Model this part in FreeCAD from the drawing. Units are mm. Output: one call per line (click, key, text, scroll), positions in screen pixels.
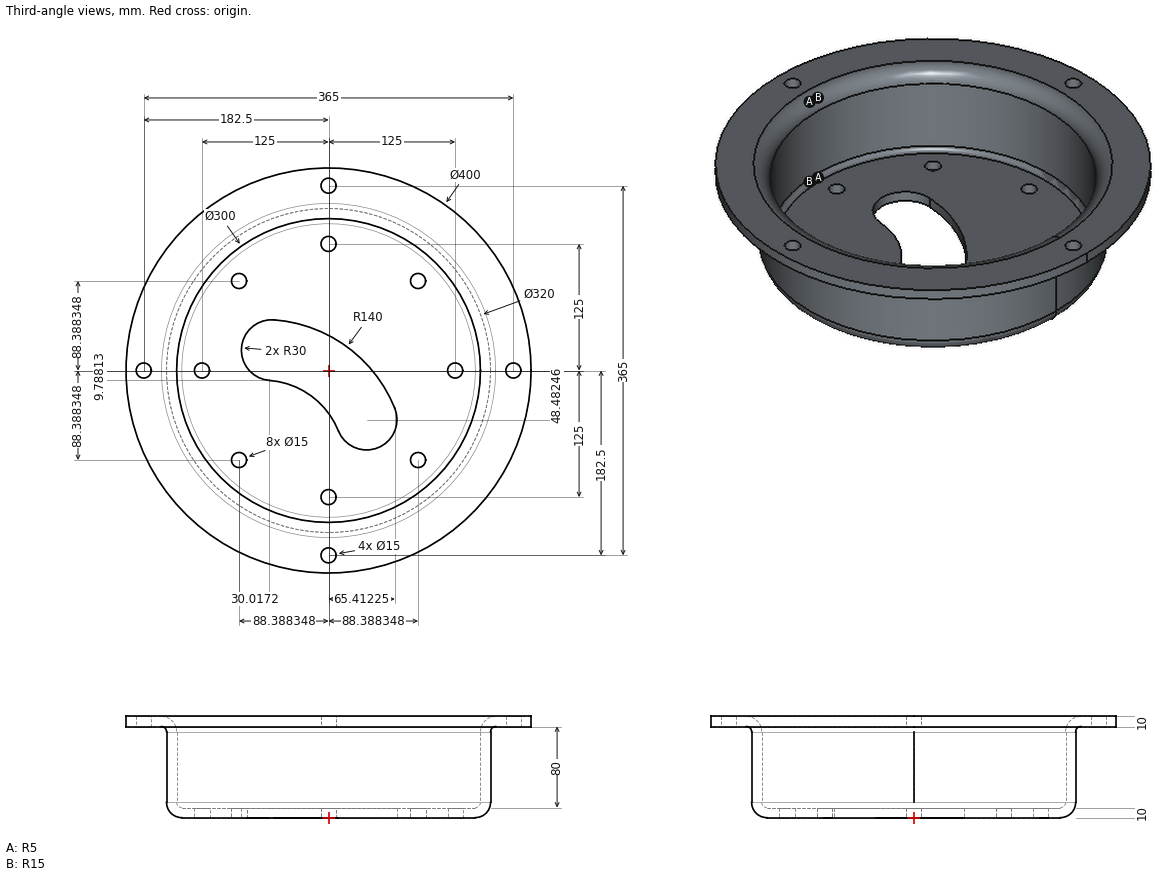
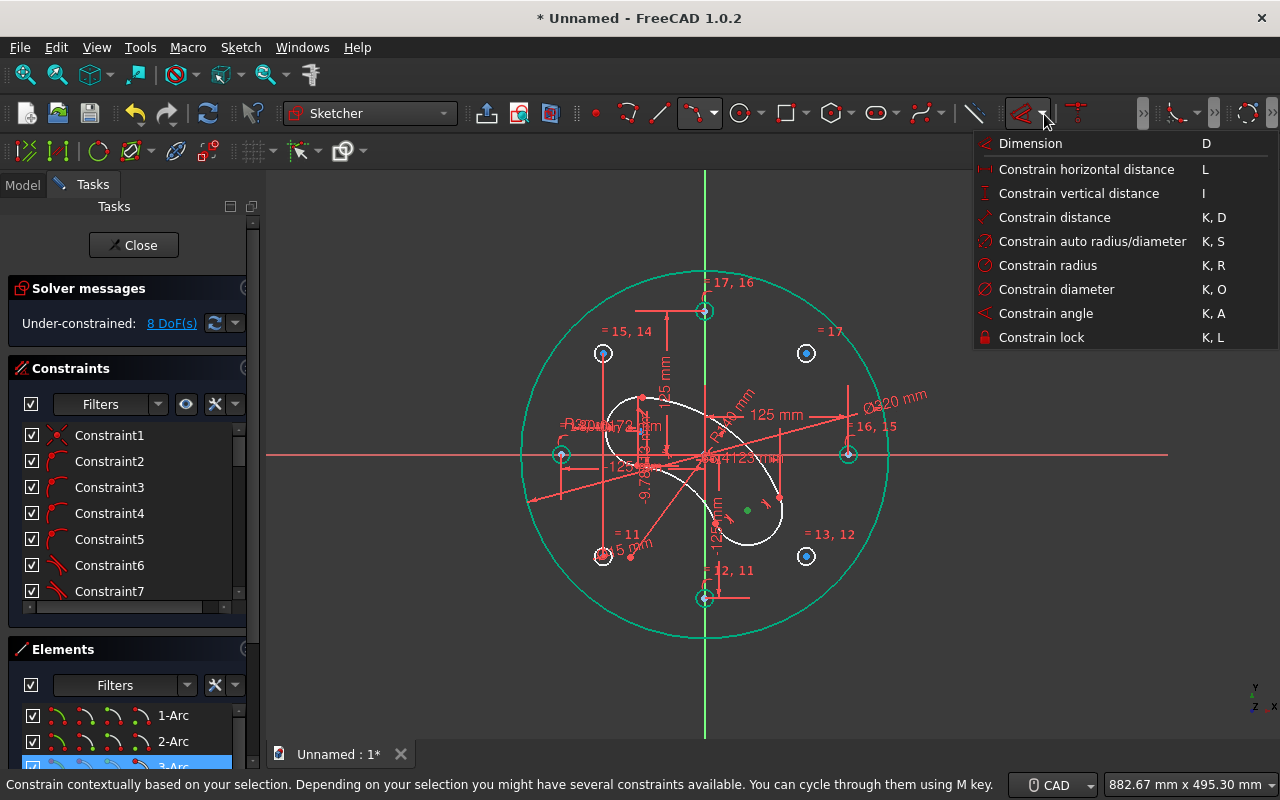
click(1126, 193)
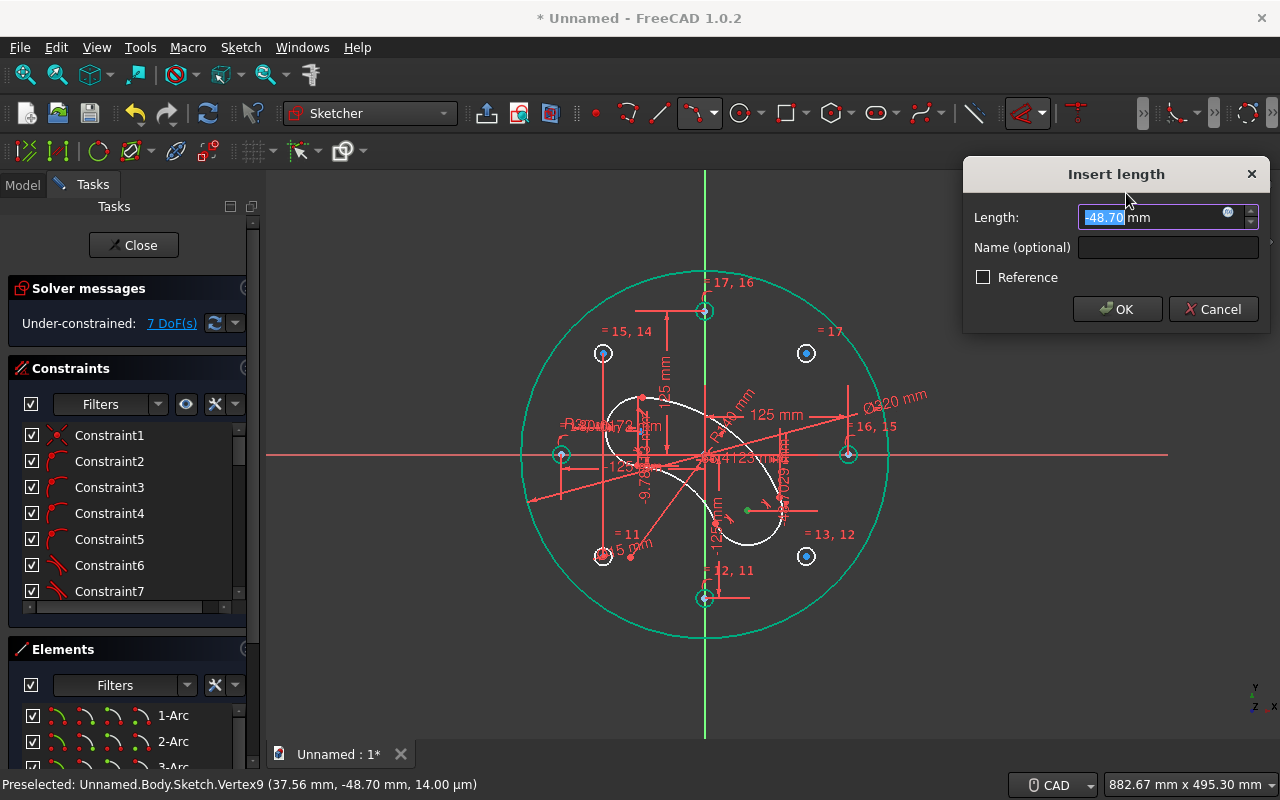
text(-48.48246)
key(Return)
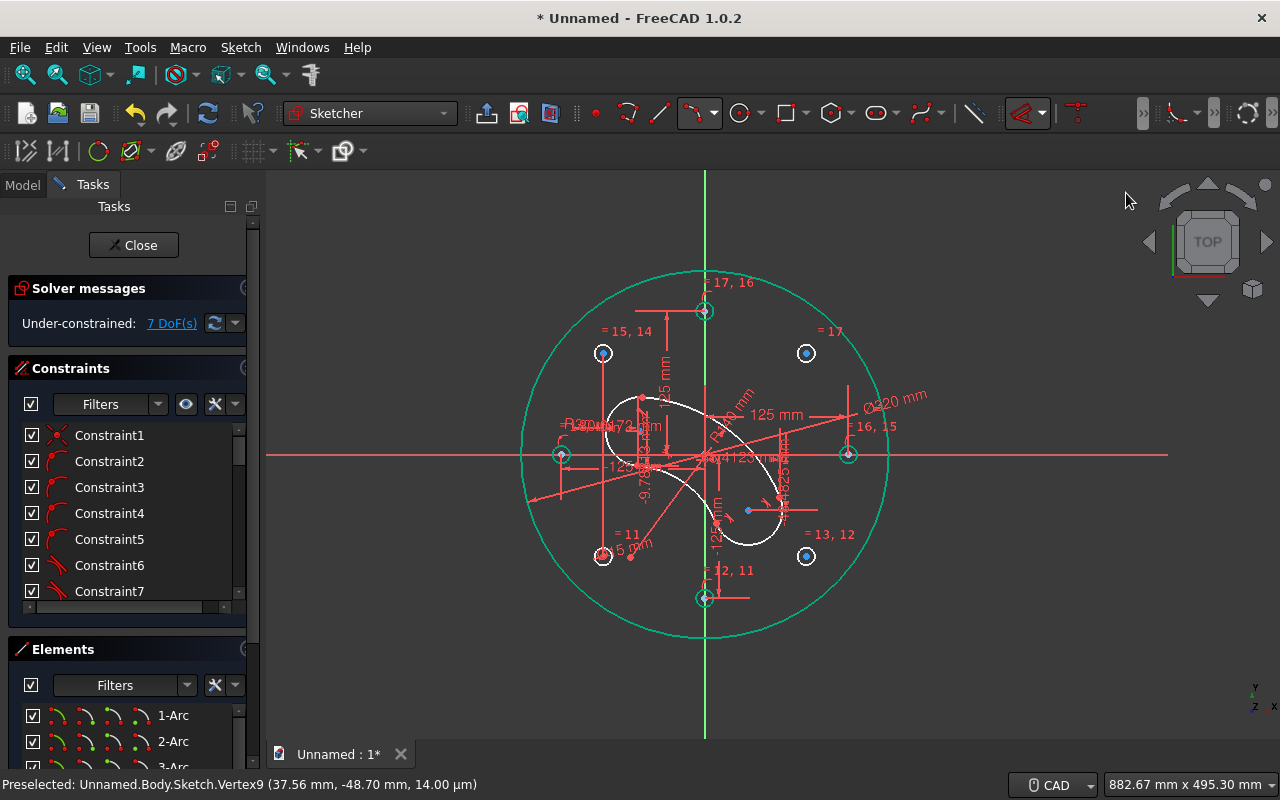
click(603, 557)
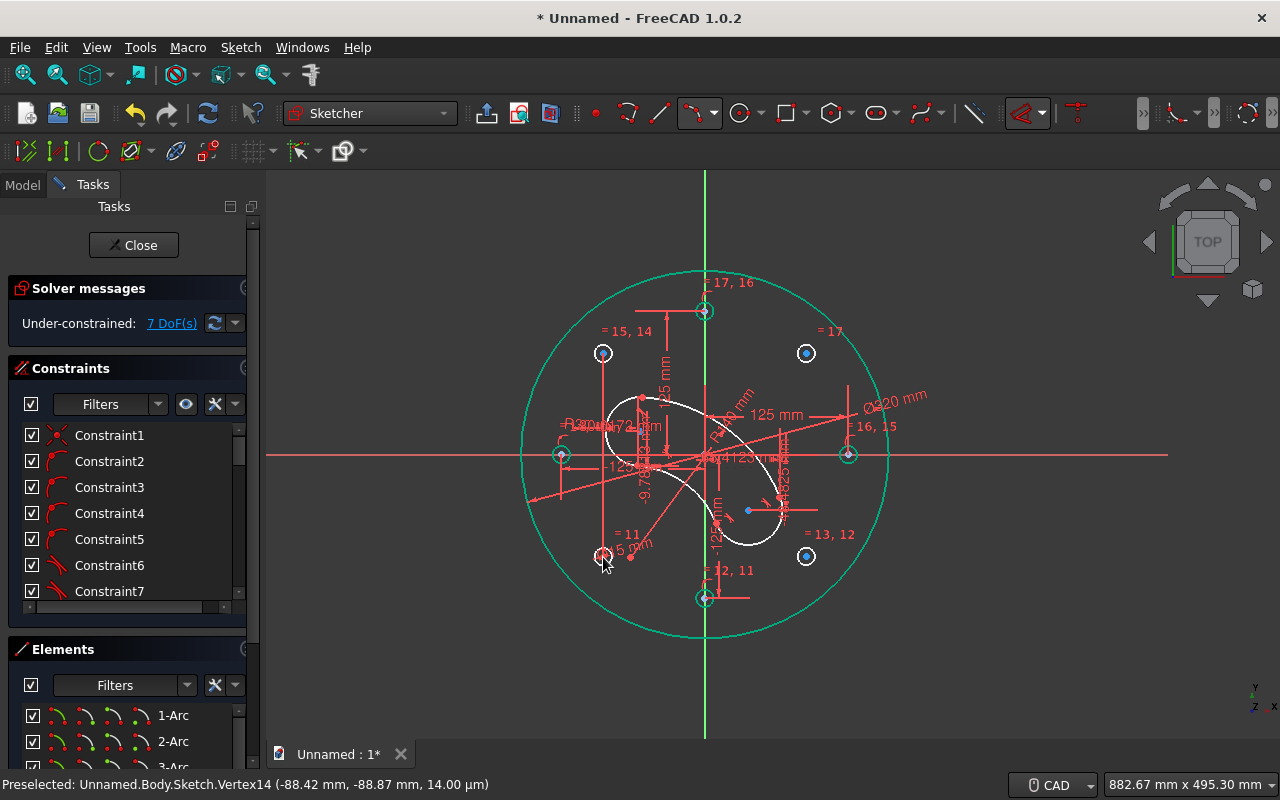
key(l)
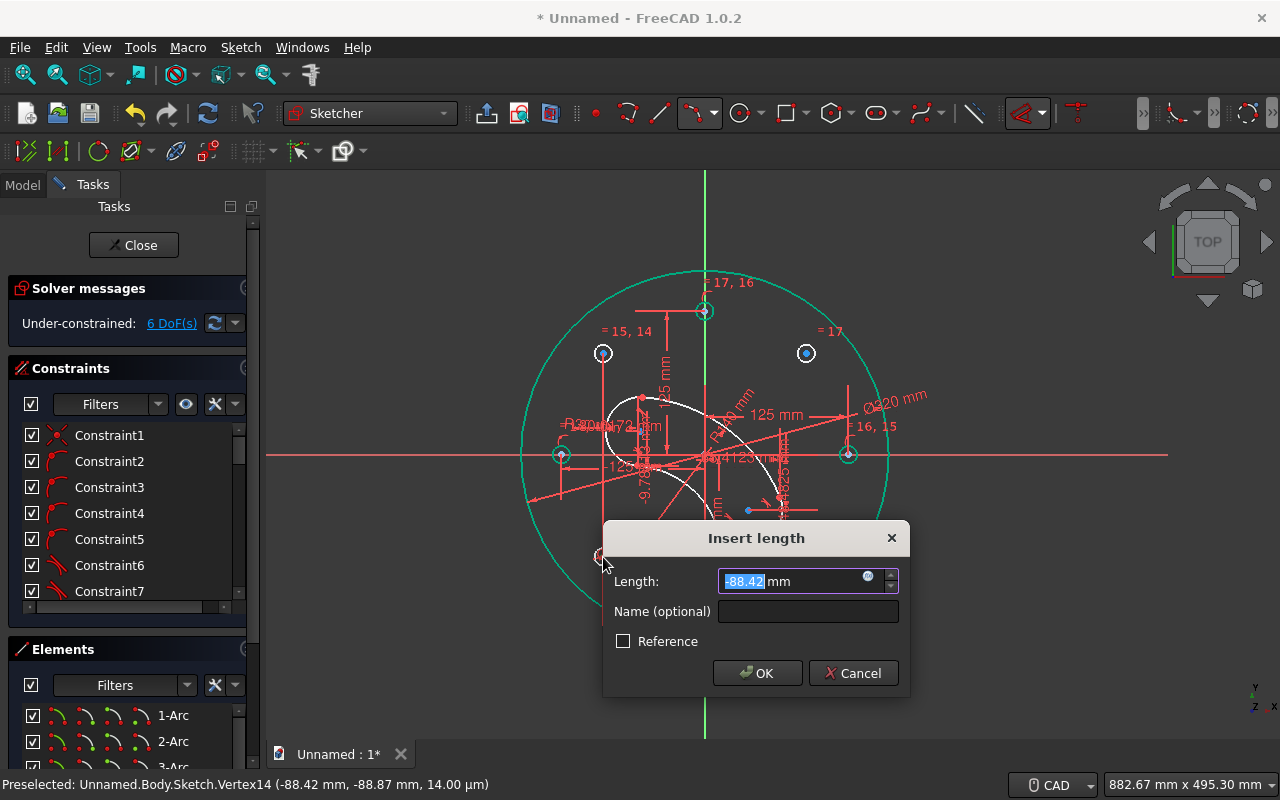
text(-88.388348)
key(Return)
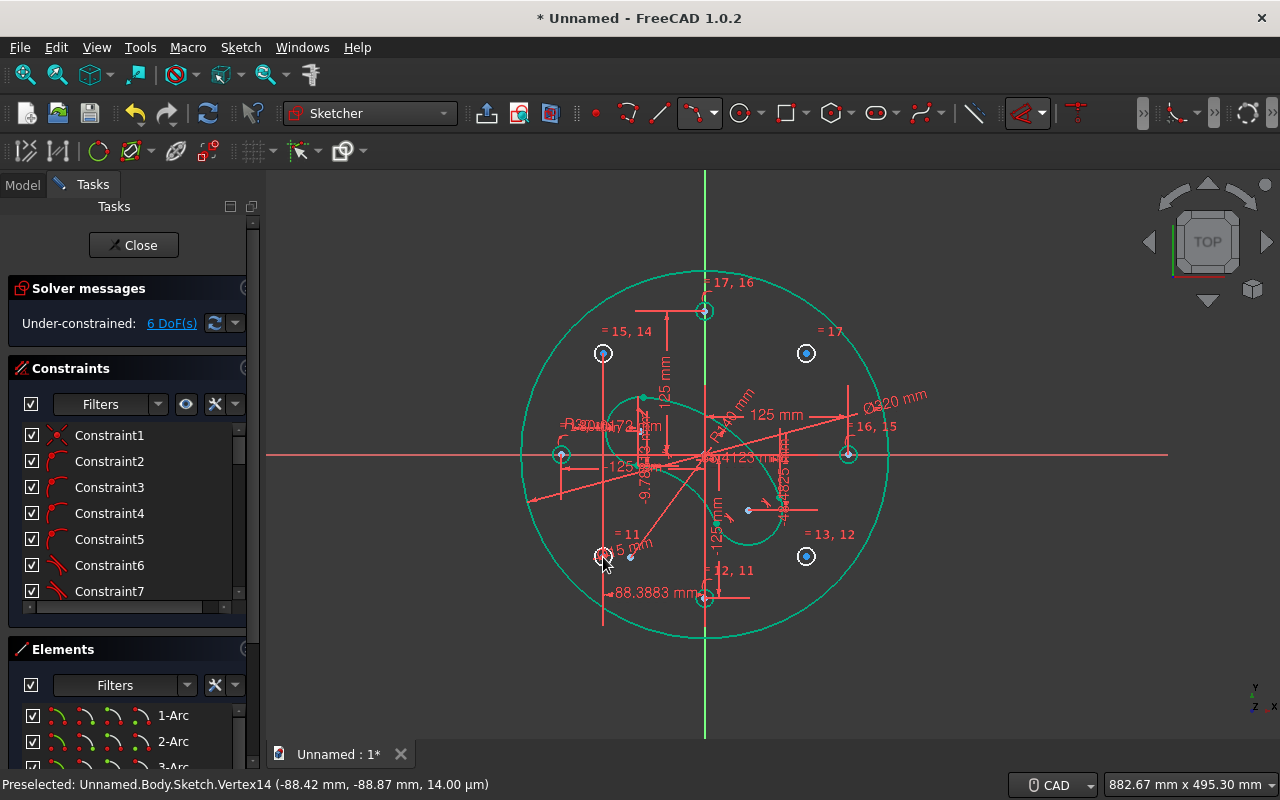
click(603, 557)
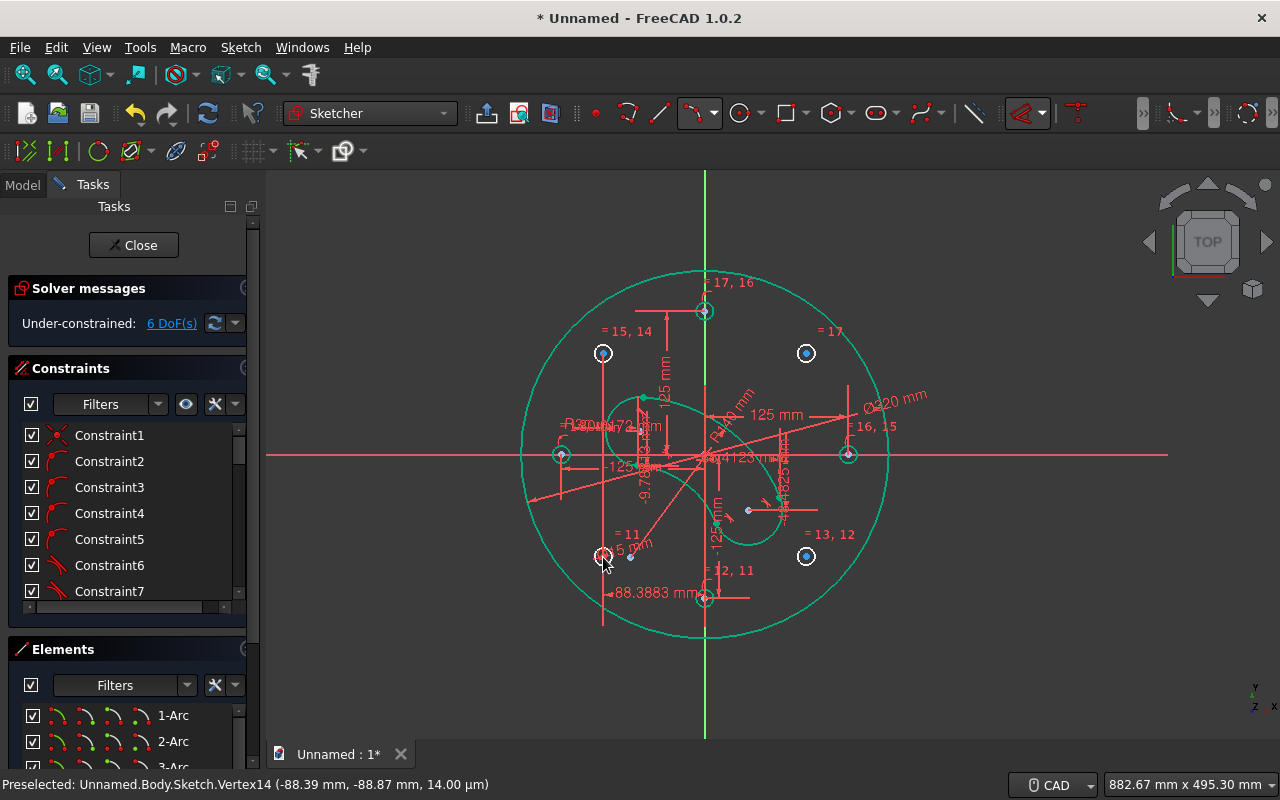
click(1044, 114)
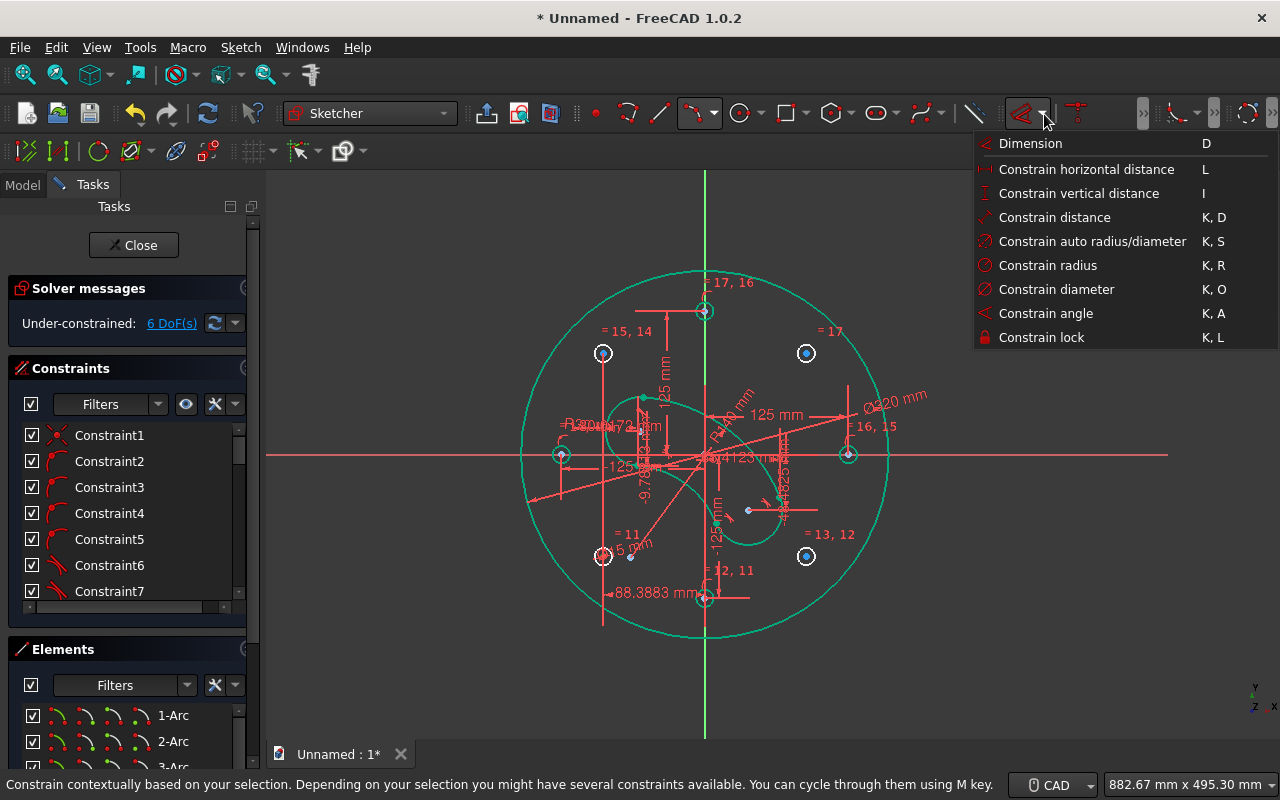
click(1126, 193)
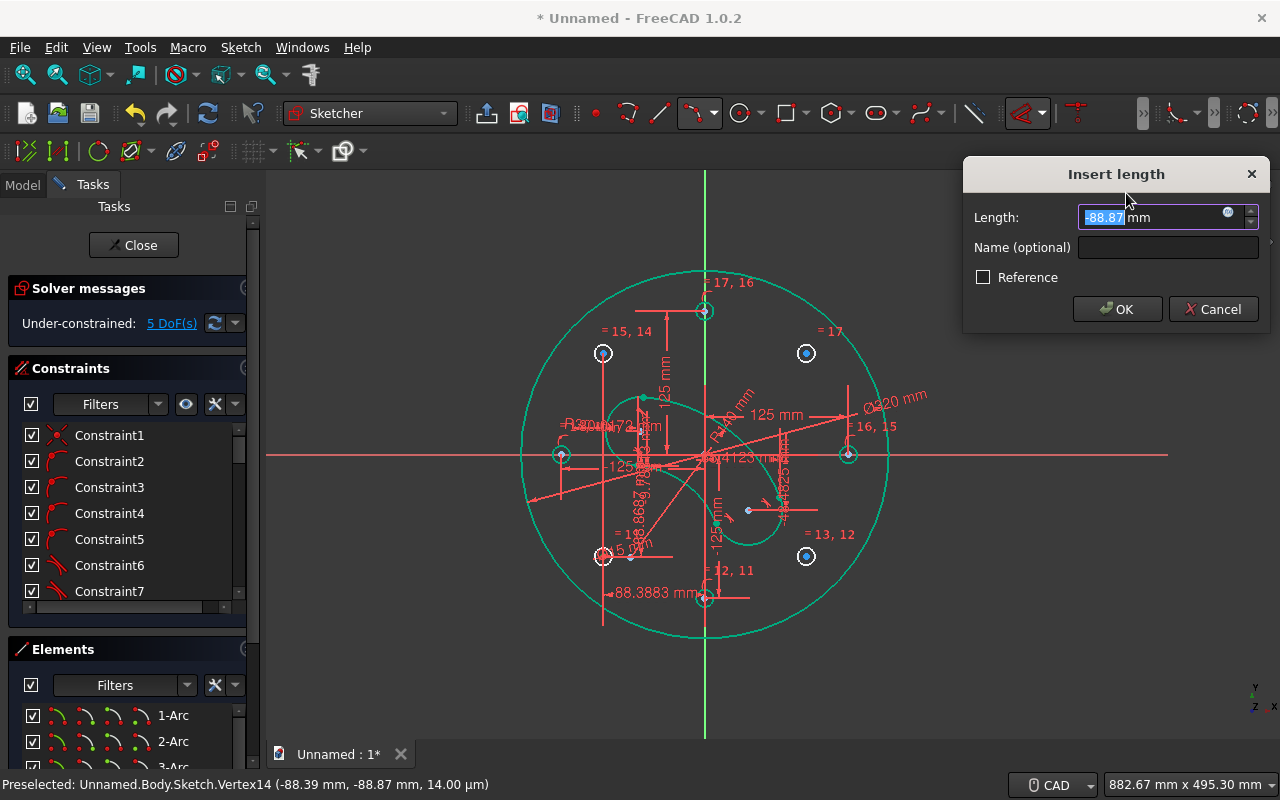
text(-88.388348)
key(Return)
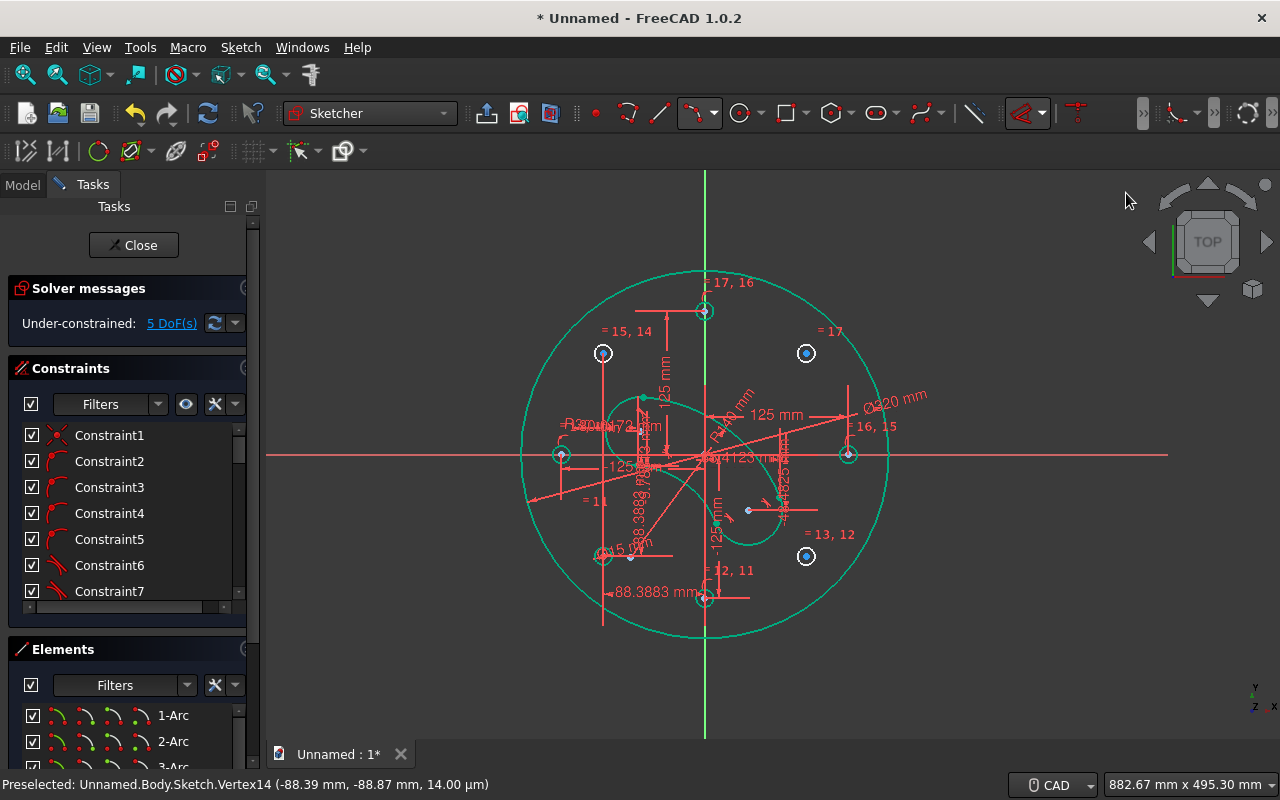
click(806, 556)